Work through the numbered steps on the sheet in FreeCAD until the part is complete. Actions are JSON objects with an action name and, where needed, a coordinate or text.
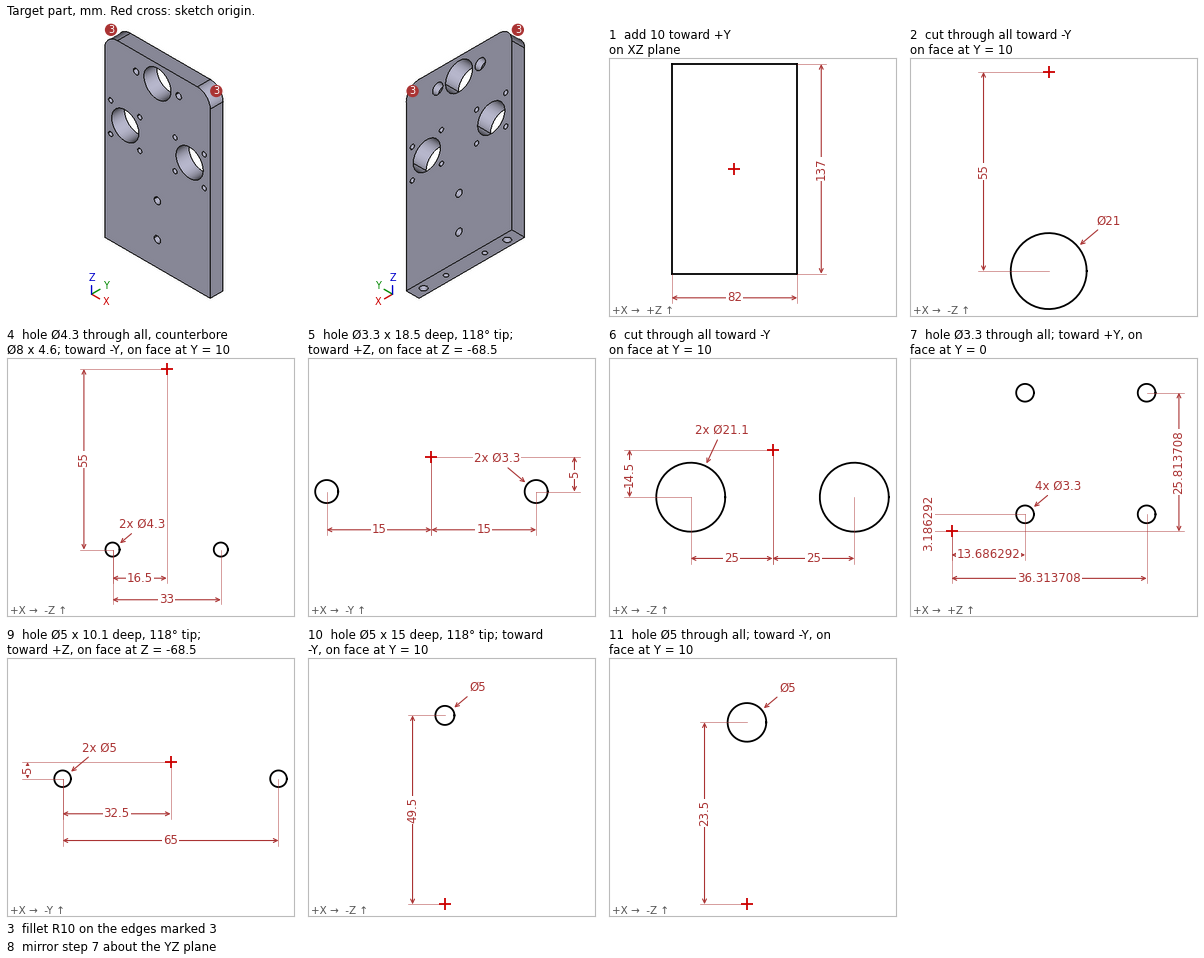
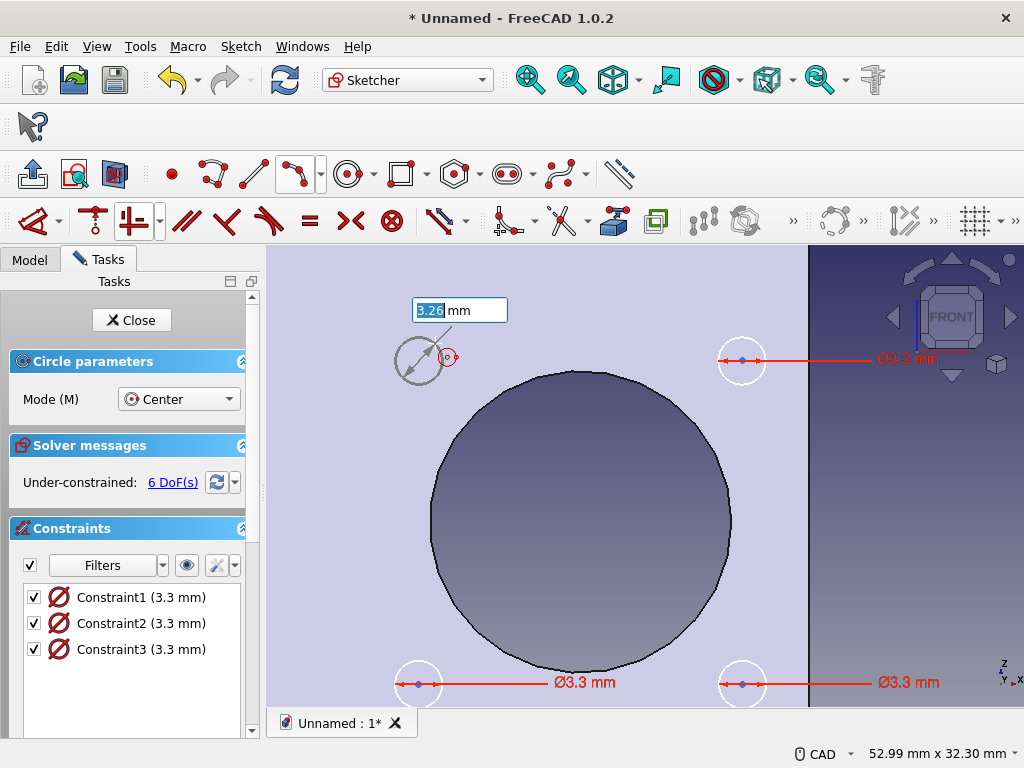
{"action": "type", "text": "3.3"}
{"action": "key", "text": "Return"}
{"action": "key", "text": "Escape"}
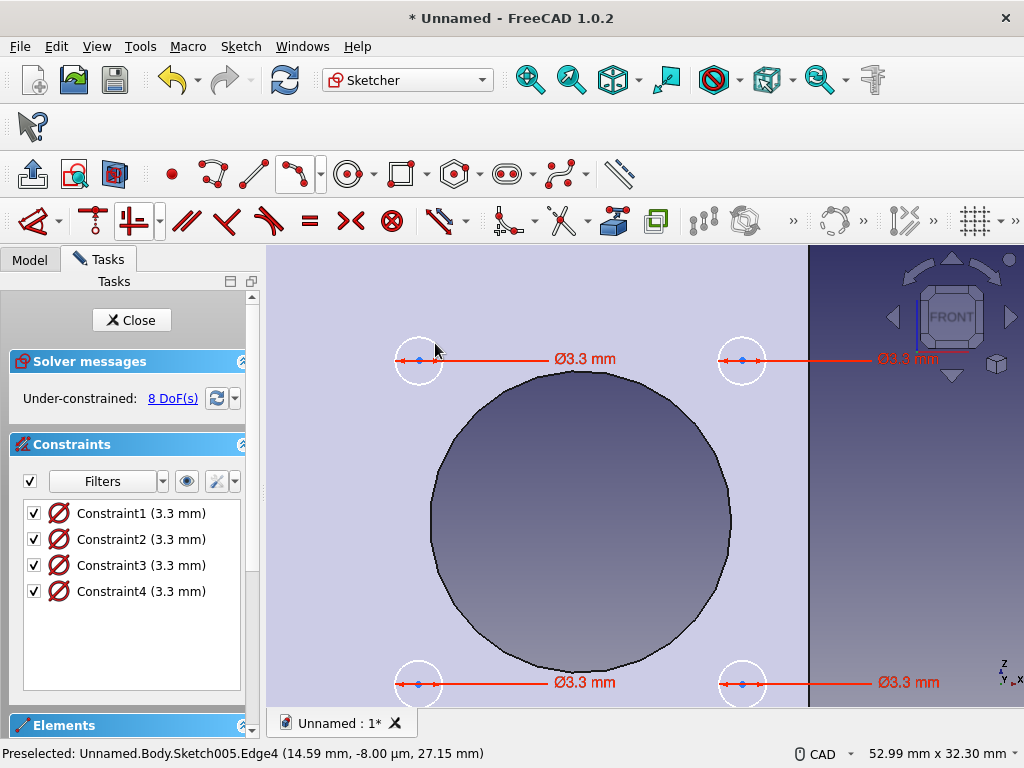
{"action": "scroll", "coordinate": [743, 360], "scroll_direction": "down", "scroll_amount": 2}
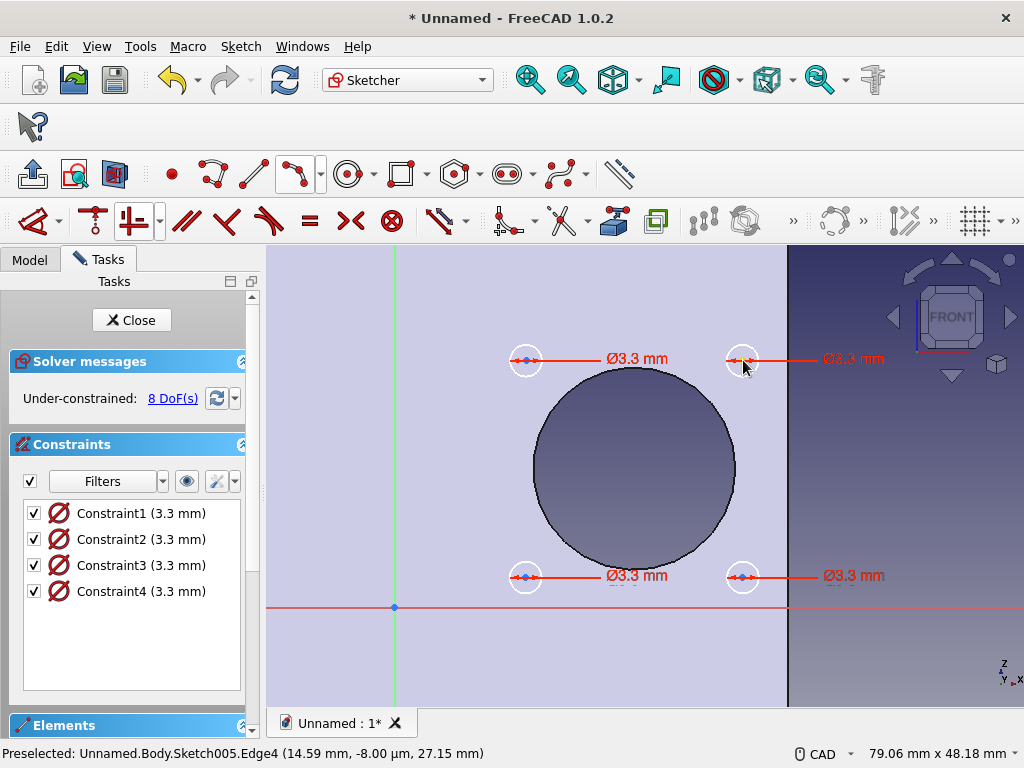
{"action": "left_click", "coordinate": [526, 578]}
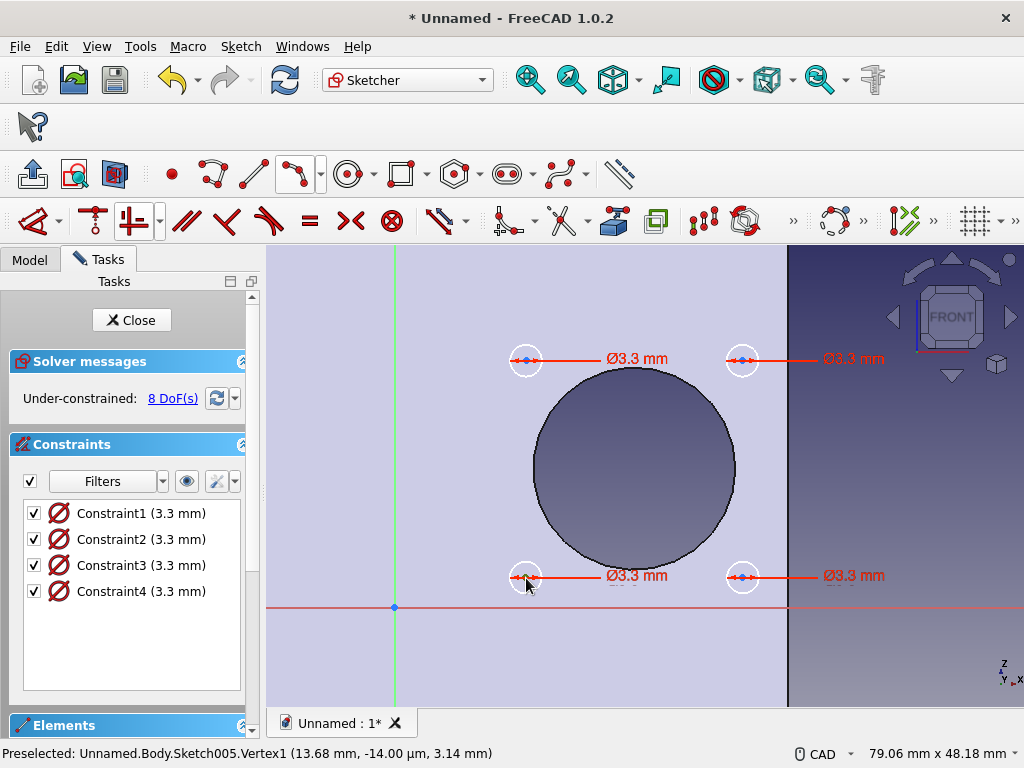
{"action": "left_click", "coordinate": [743, 578]}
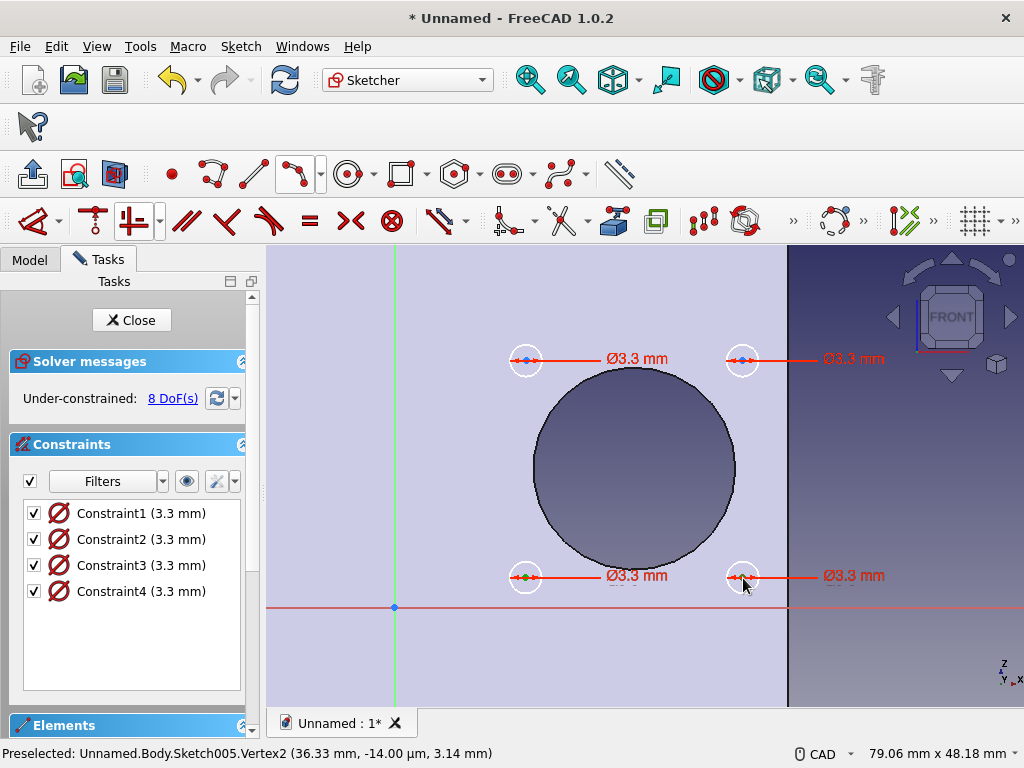
{"action": "key", "text": "h"}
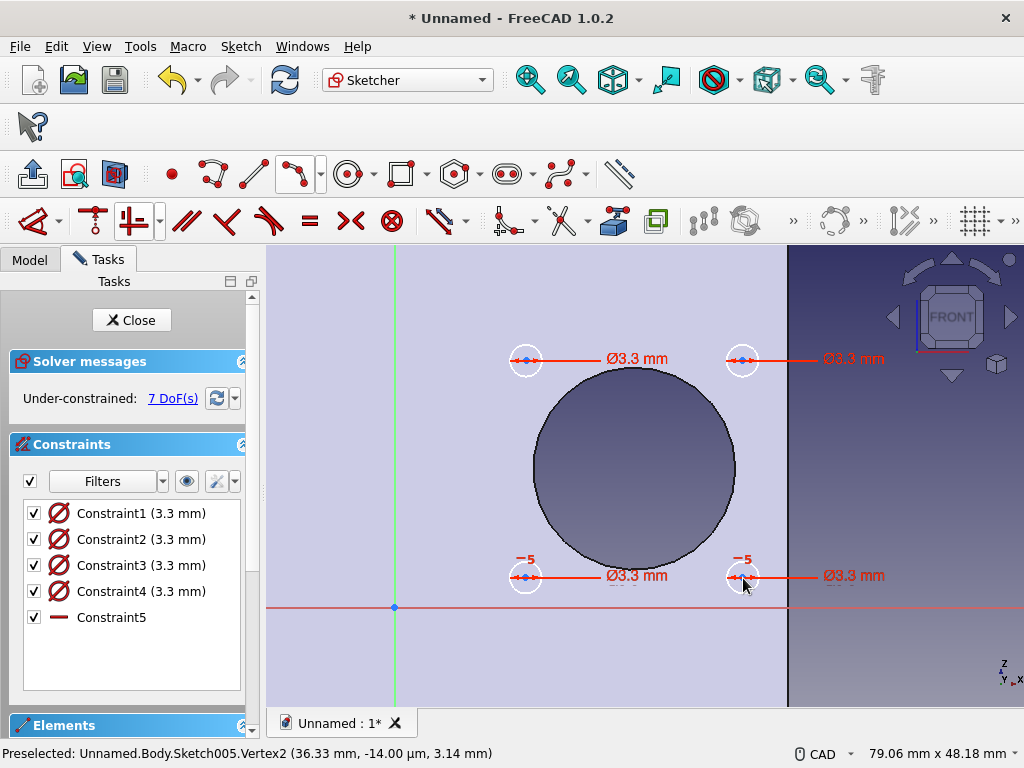
{"action": "left_click", "coordinate": [743, 578]}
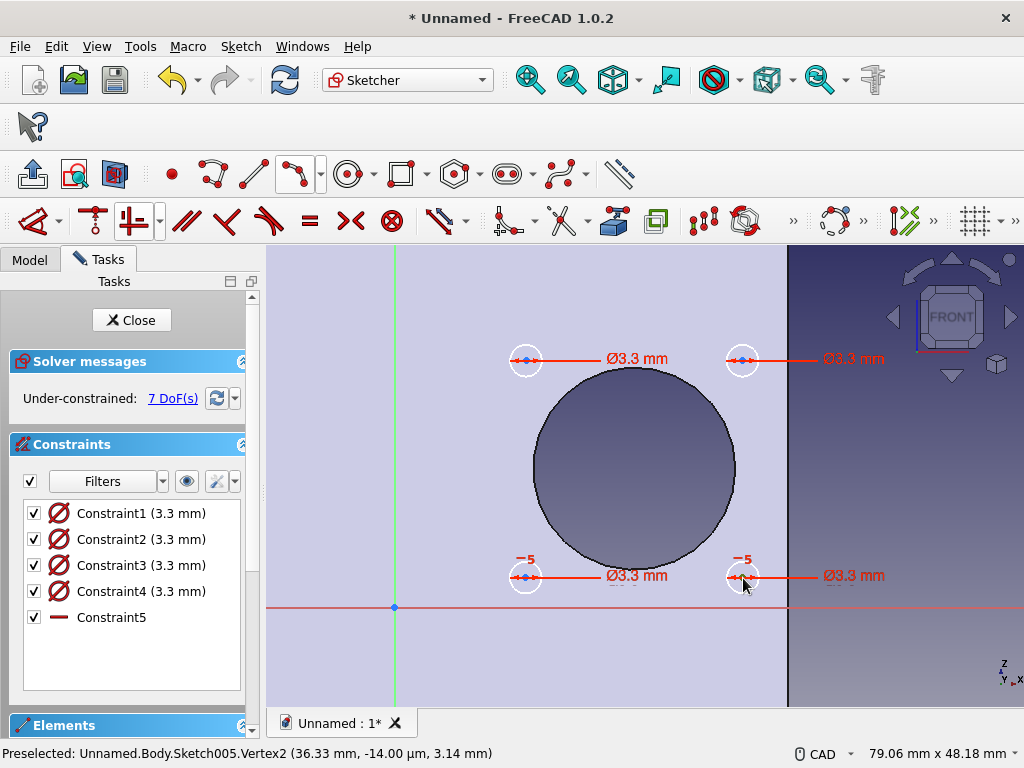
{"action": "left_click", "coordinate": [743, 361]}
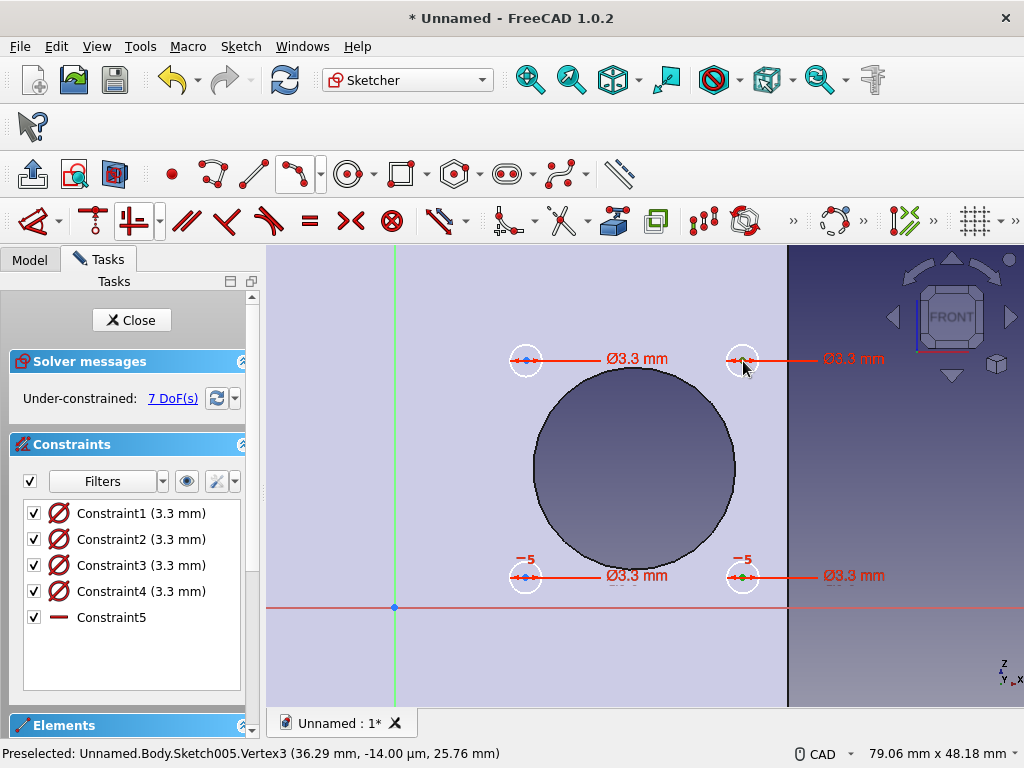
{"action": "key", "text": "v"}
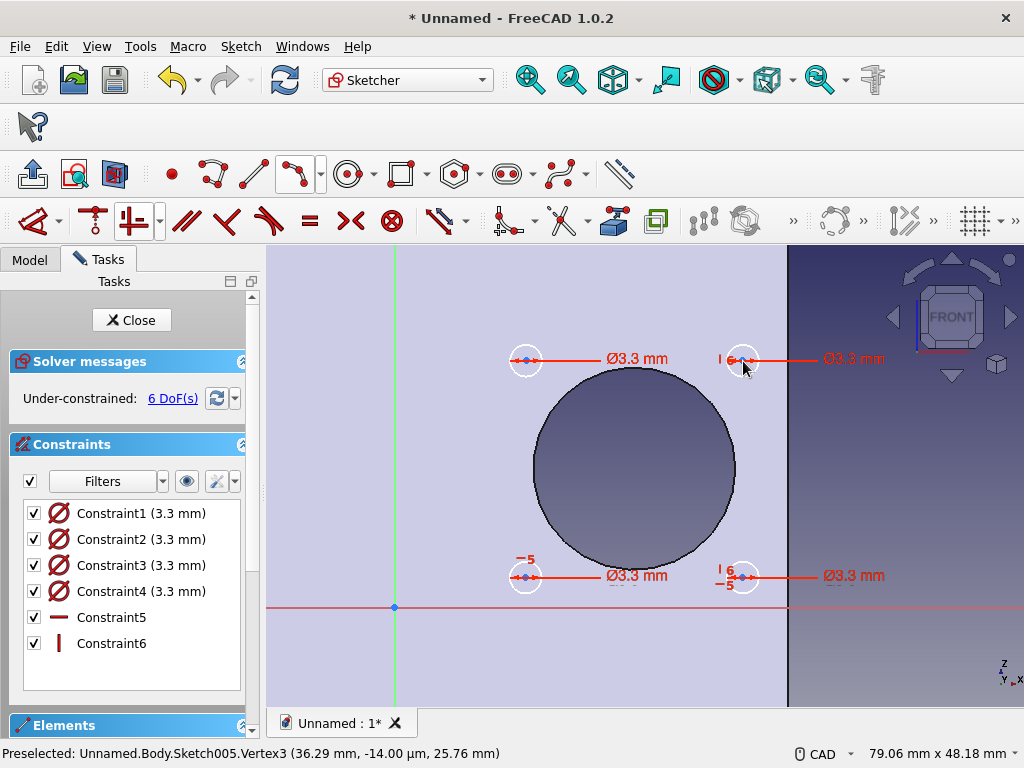
{"action": "left_click", "coordinate": [526, 578]}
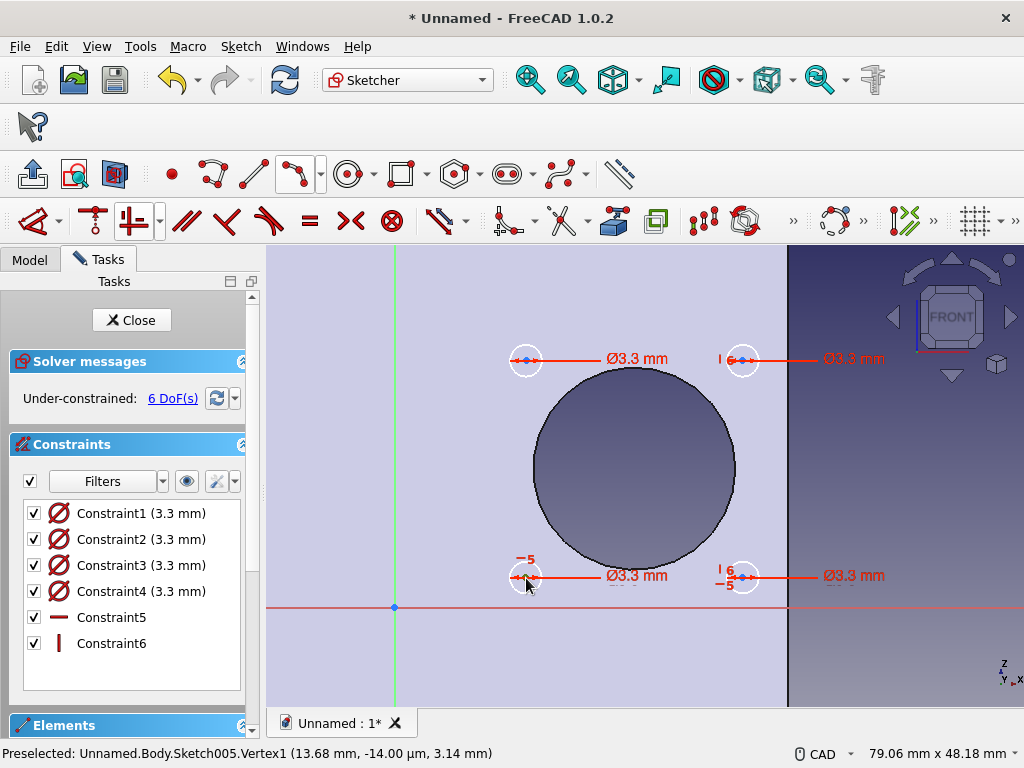
{"action": "left_click", "coordinate": [526, 361]}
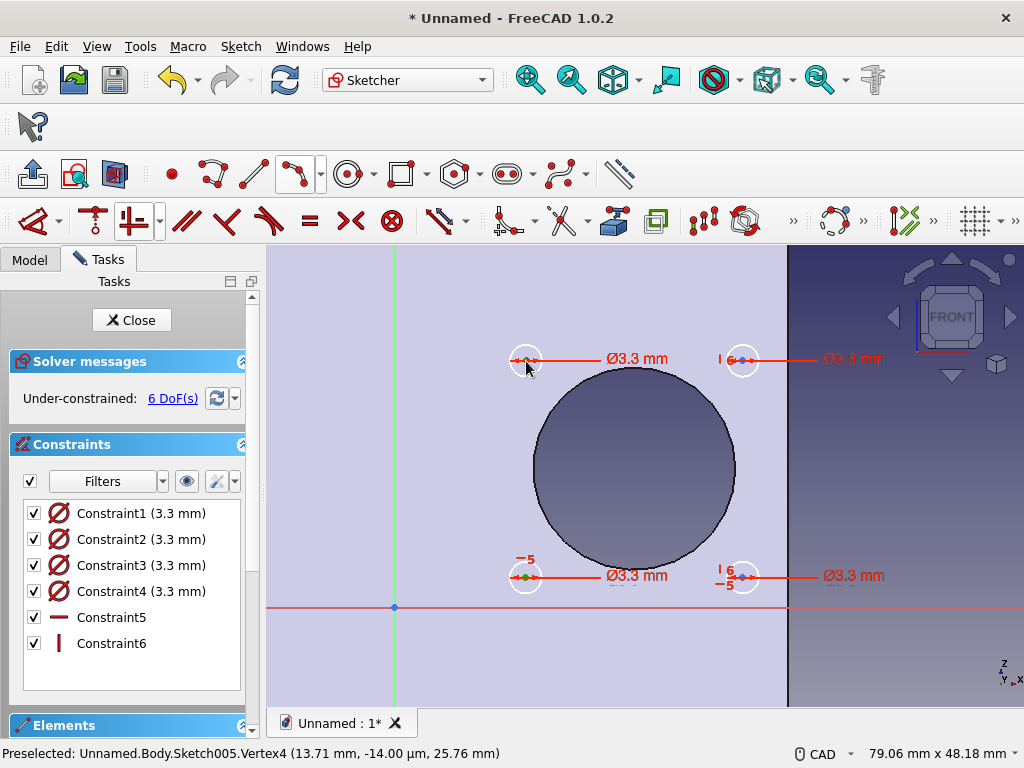
{"action": "key", "text": "v"}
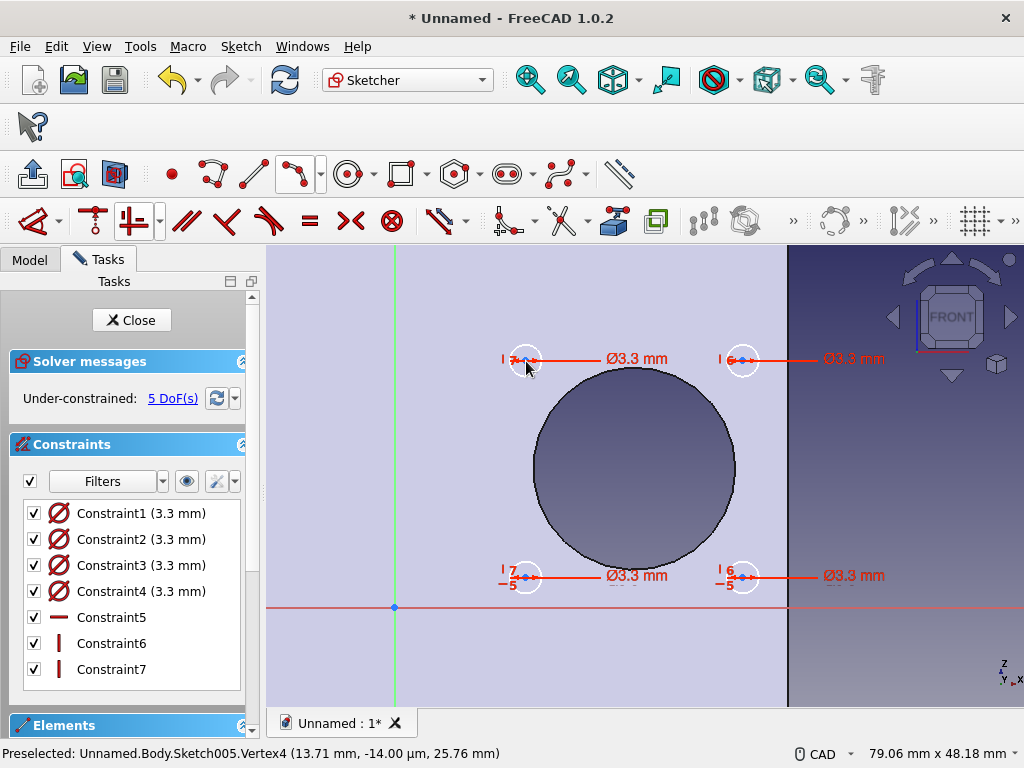
{"action": "left_click", "coordinate": [743, 361]}